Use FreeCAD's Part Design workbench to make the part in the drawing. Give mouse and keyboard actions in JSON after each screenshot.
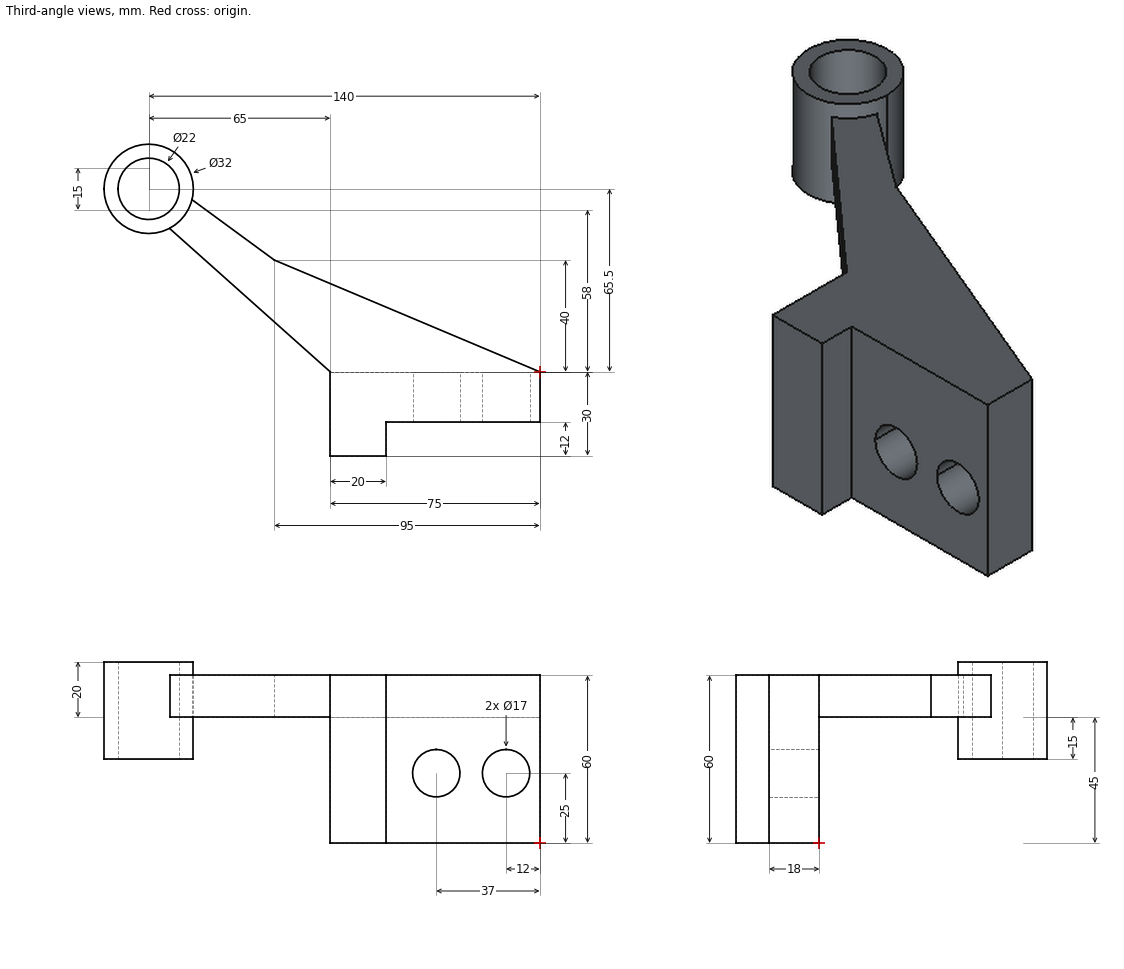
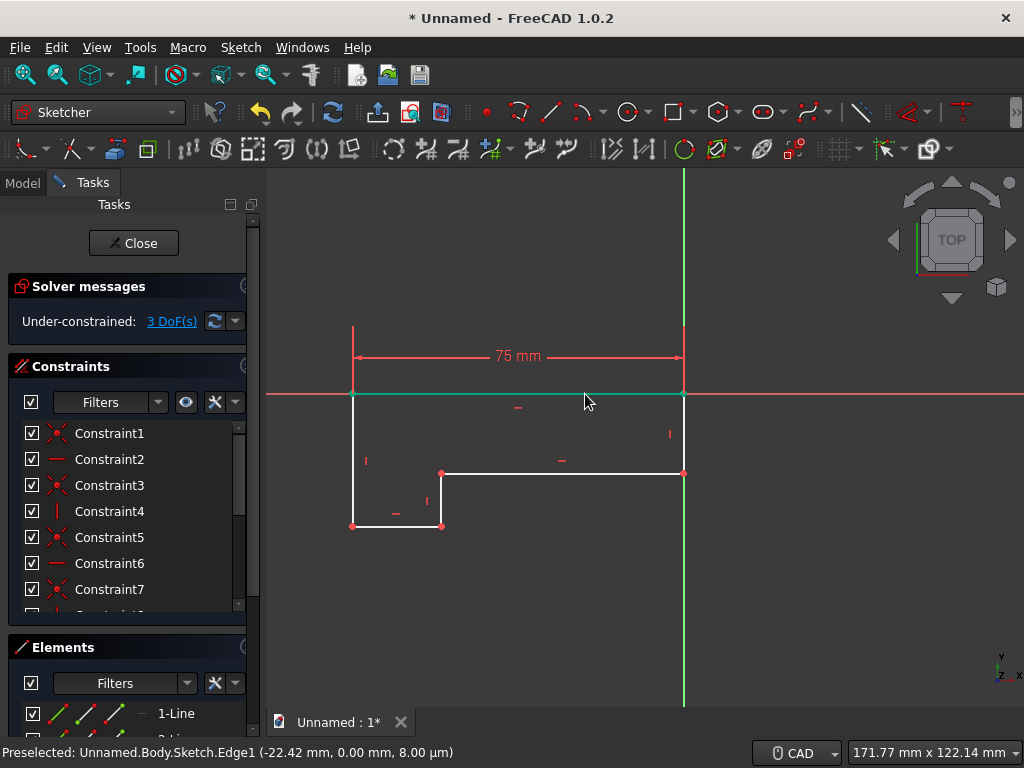
{"action": "left_click", "coordinate": [353, 434]}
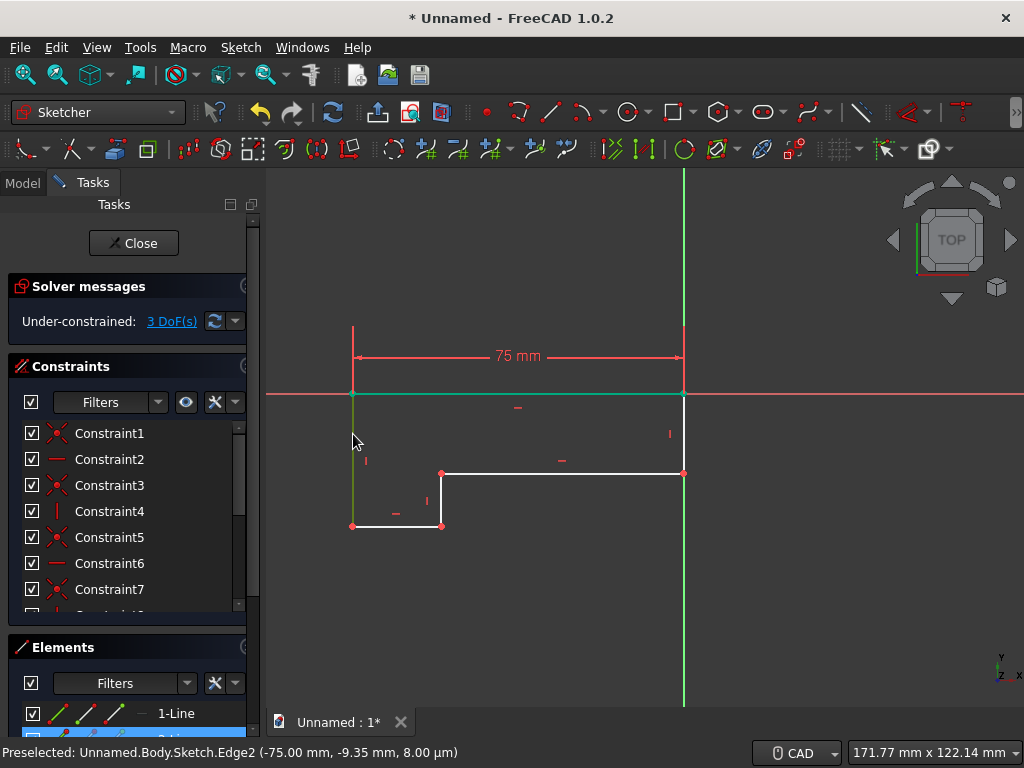
{"action": "left_click", "coordinate": [930, 112]}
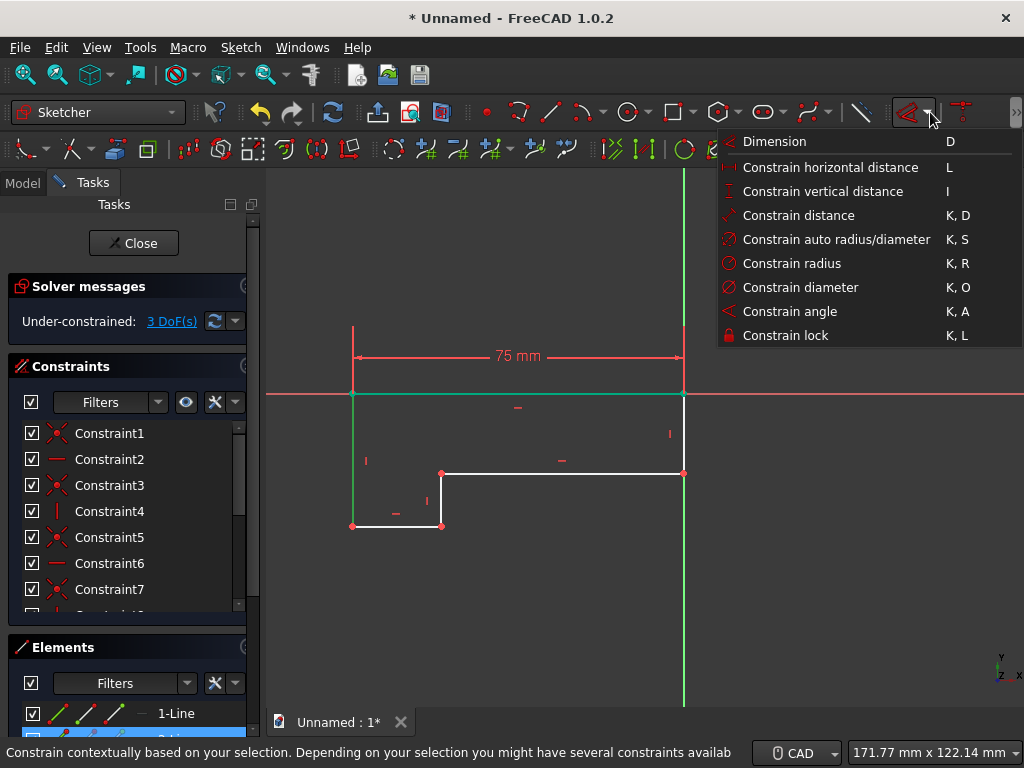
{"action": "left_click", "coordinate": [870, 191]}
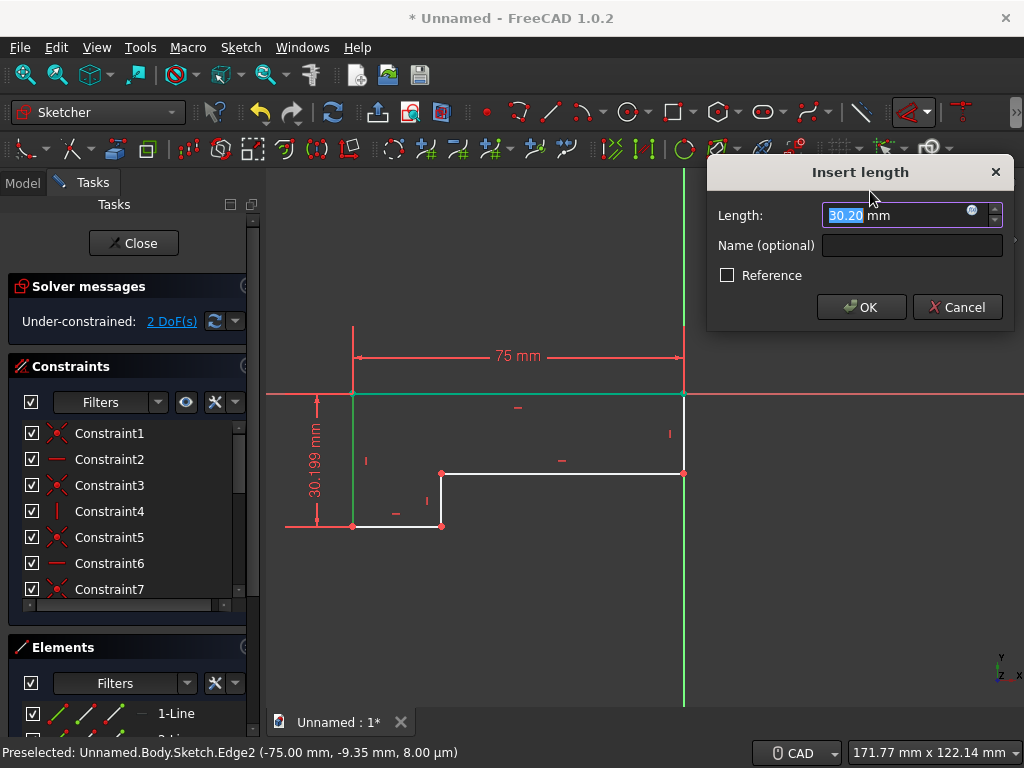
{"action": "type", "text": "30"}
{"action": "key", "text": "Return"}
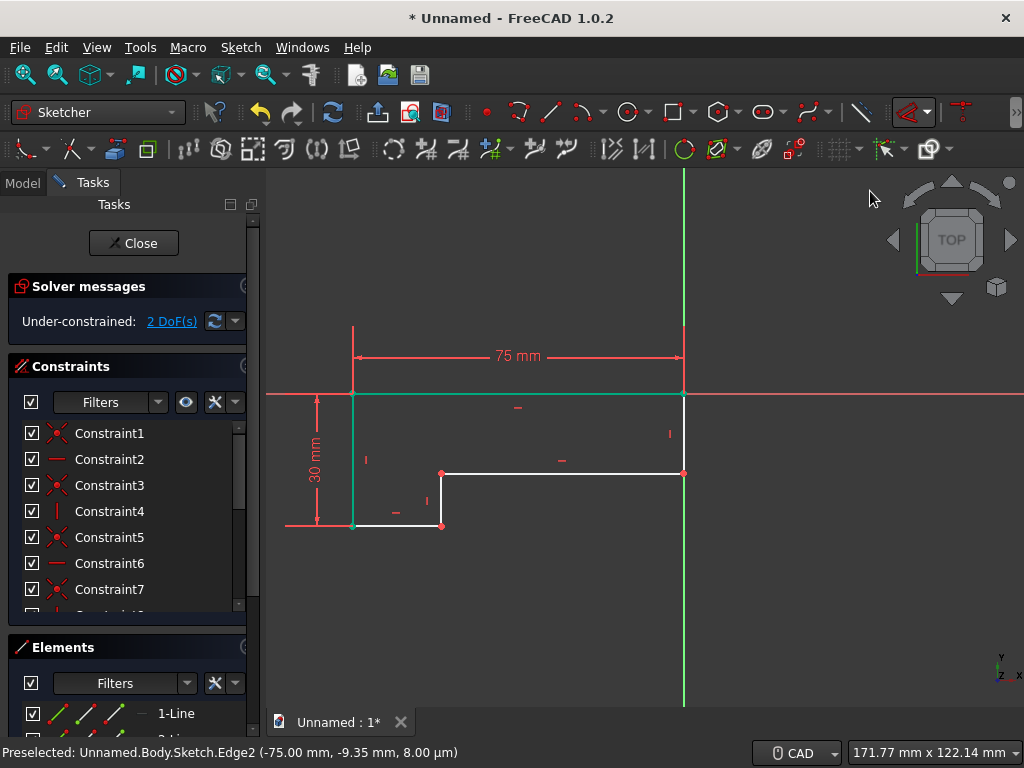
{"action": "left_click", "coordinate": [379, 526]}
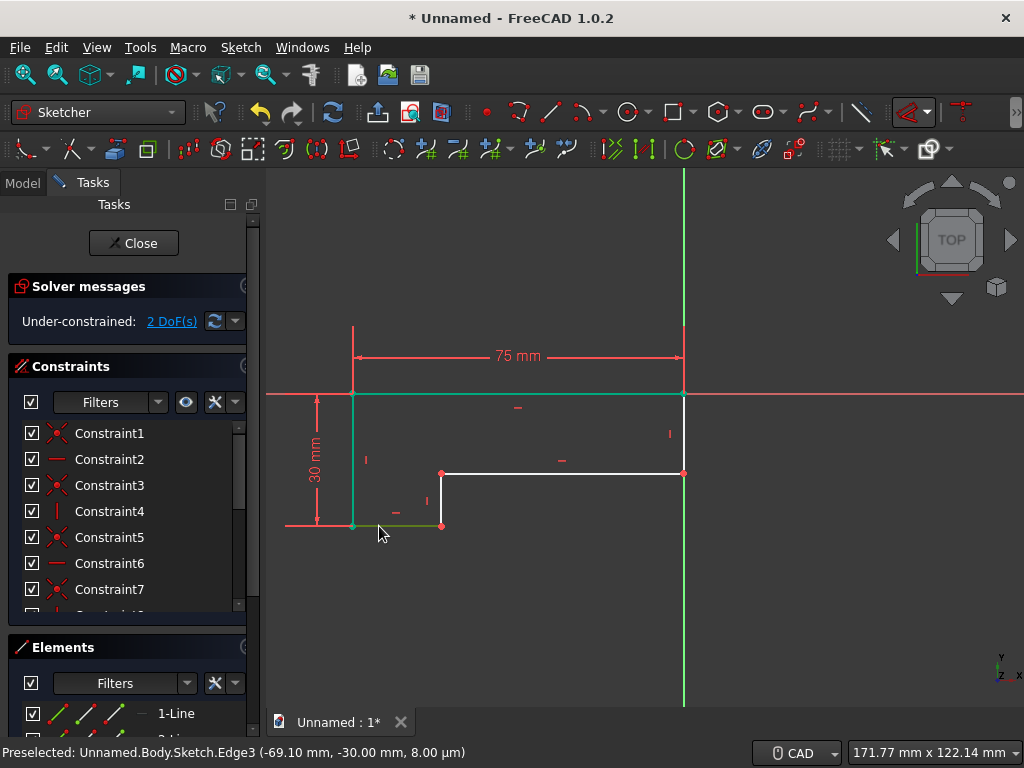
{"action": "key", "text": "l"}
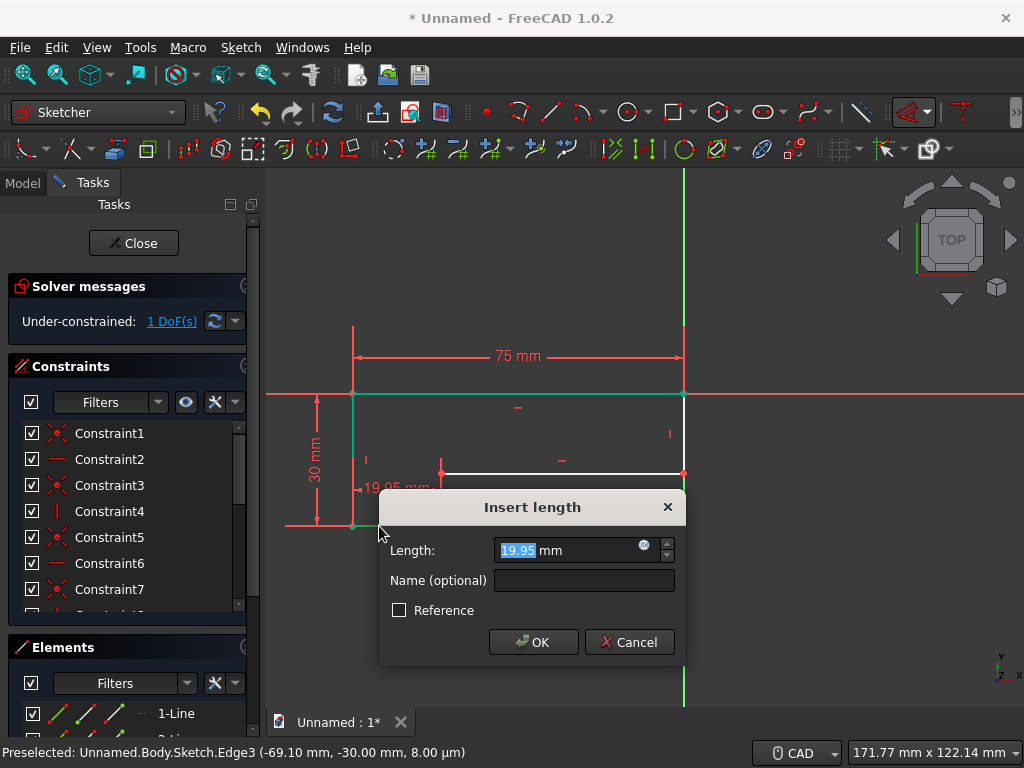
{"action": "type", "text": "20"}
{"action": "key", "text": "Return"}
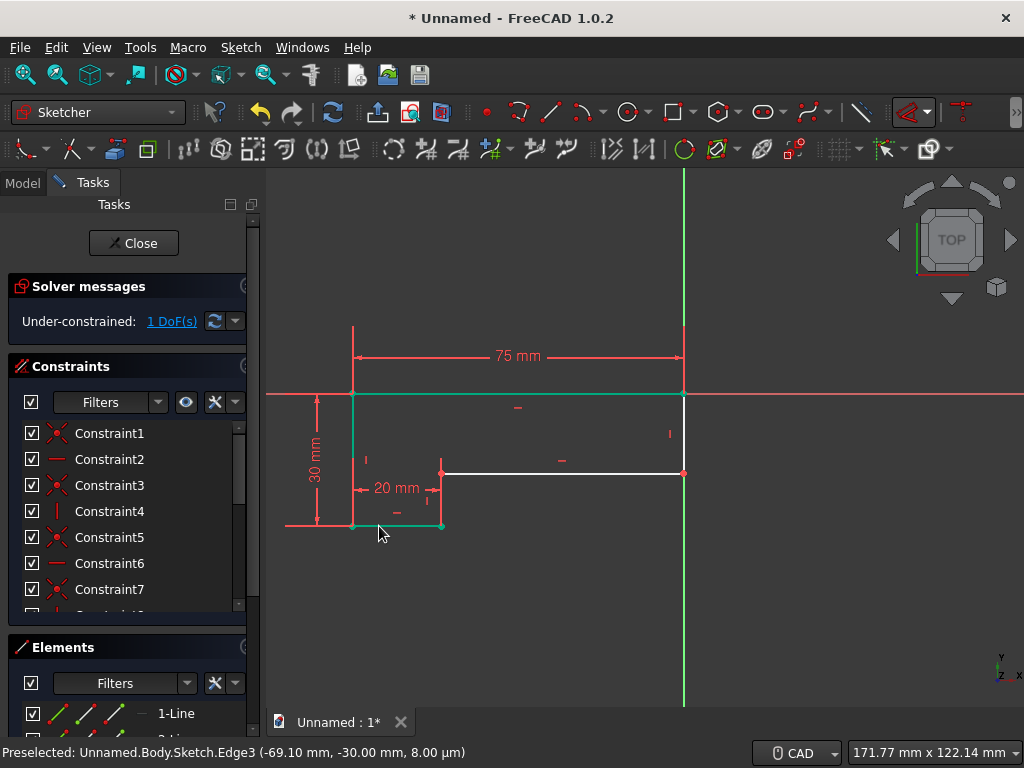
{"action": "left_click", "coordinate": [441, 510]}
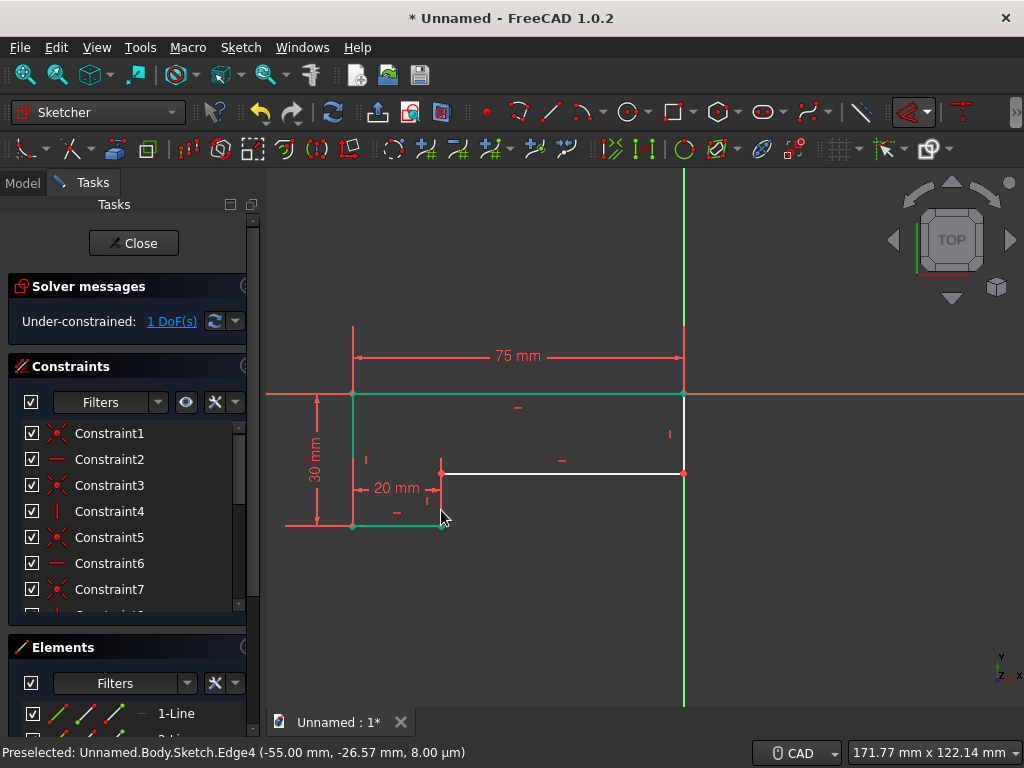
{"action": "left_click", "coordinate": [930, 112]}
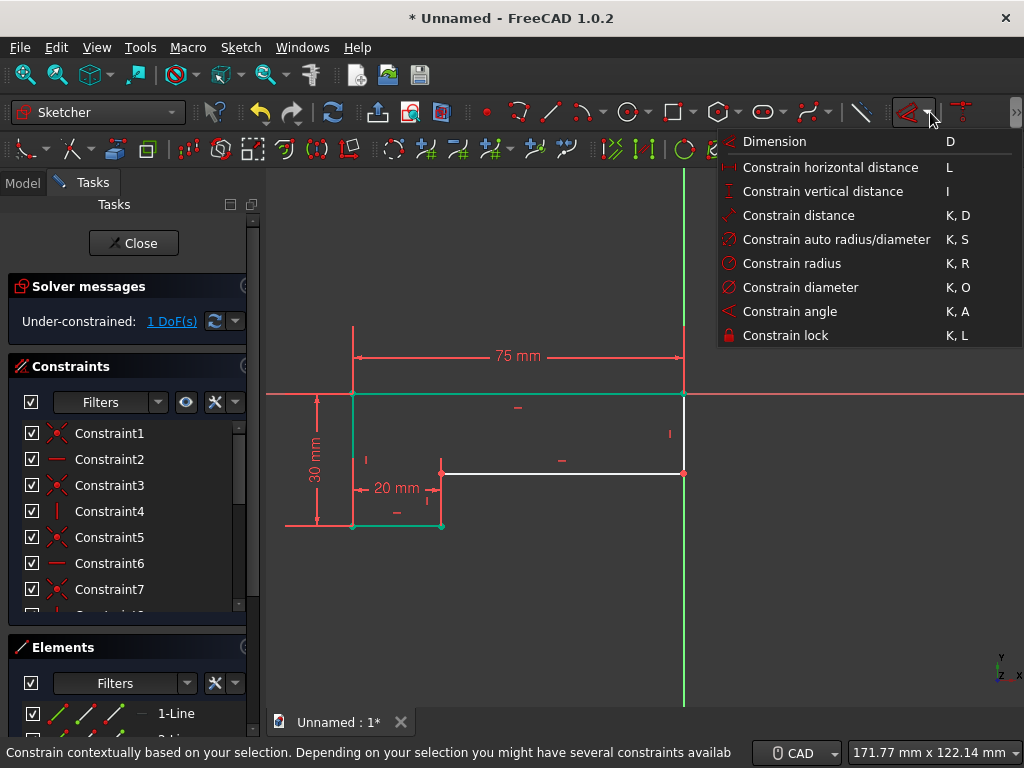
{"action": "left_click", "coordinate": [870, 191]}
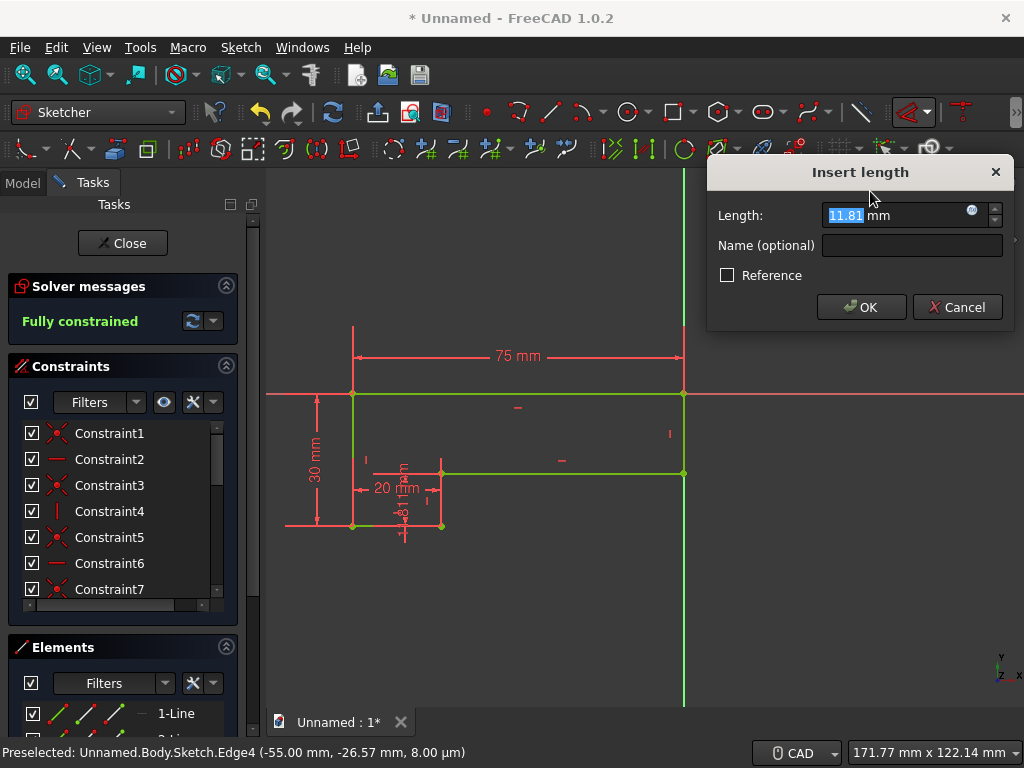
{"action": "type", "text": "12"}
{"action": "key", "text": "Return"}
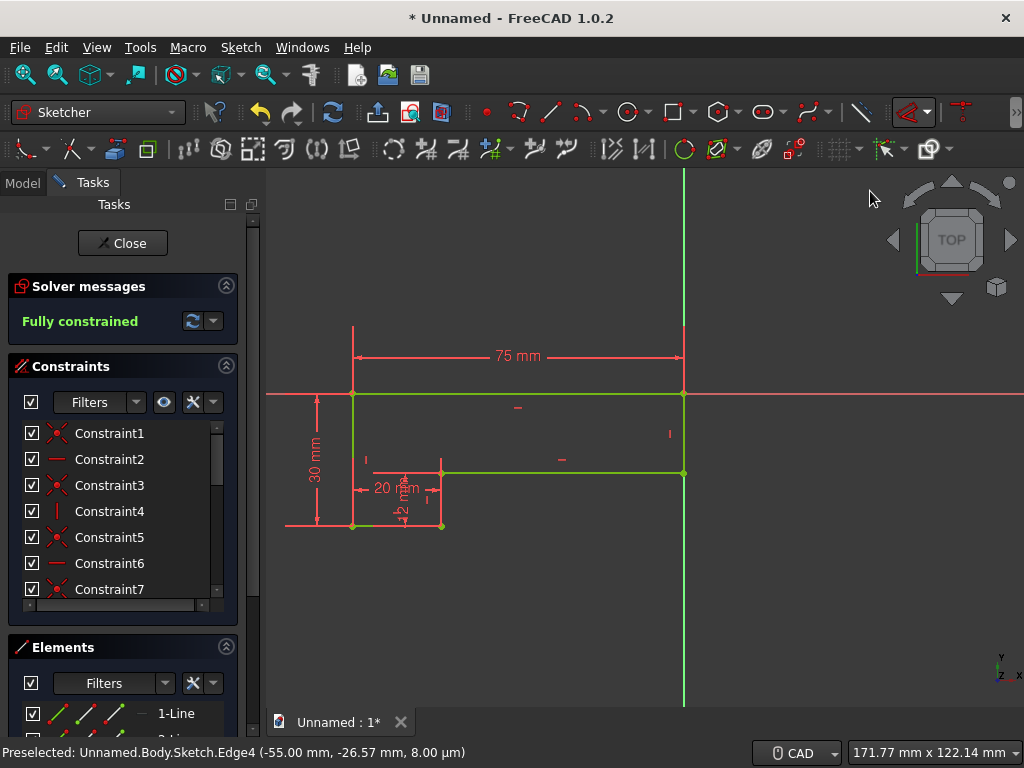
{"action": "left_click", "coordinate": [123, 243]}